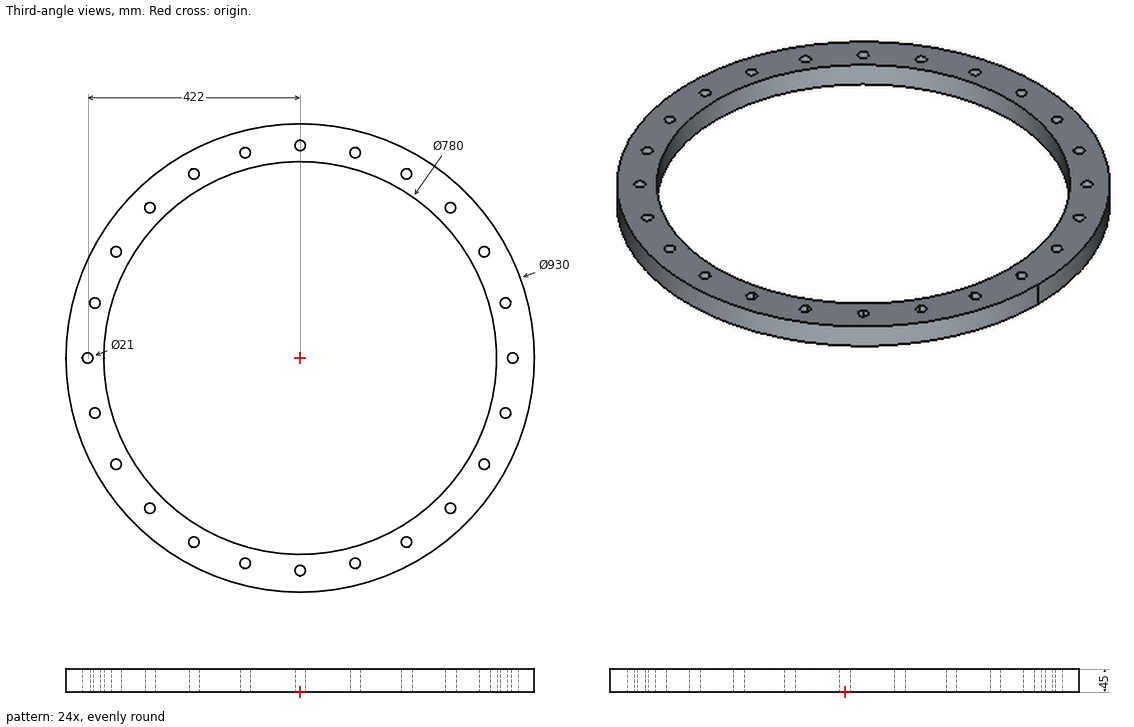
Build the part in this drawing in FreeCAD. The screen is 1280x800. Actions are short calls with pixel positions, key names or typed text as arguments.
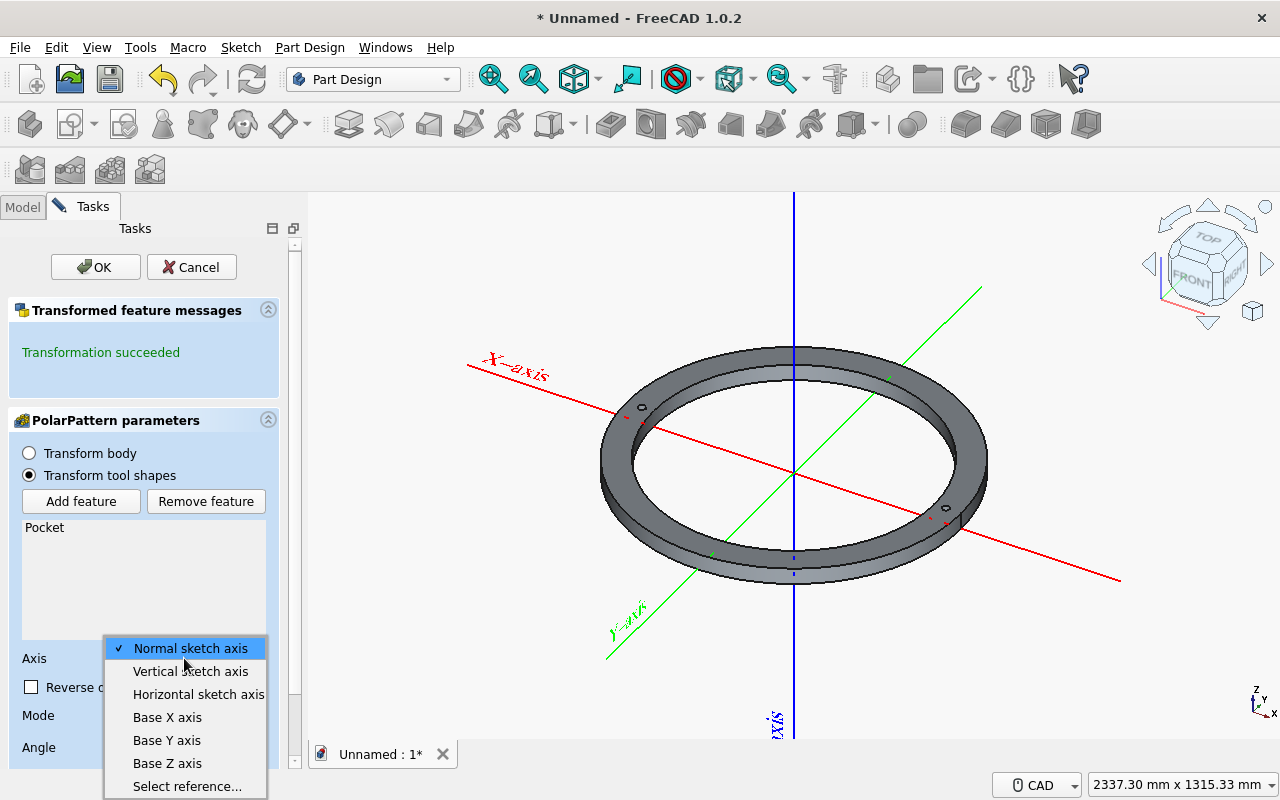
click(184, 764)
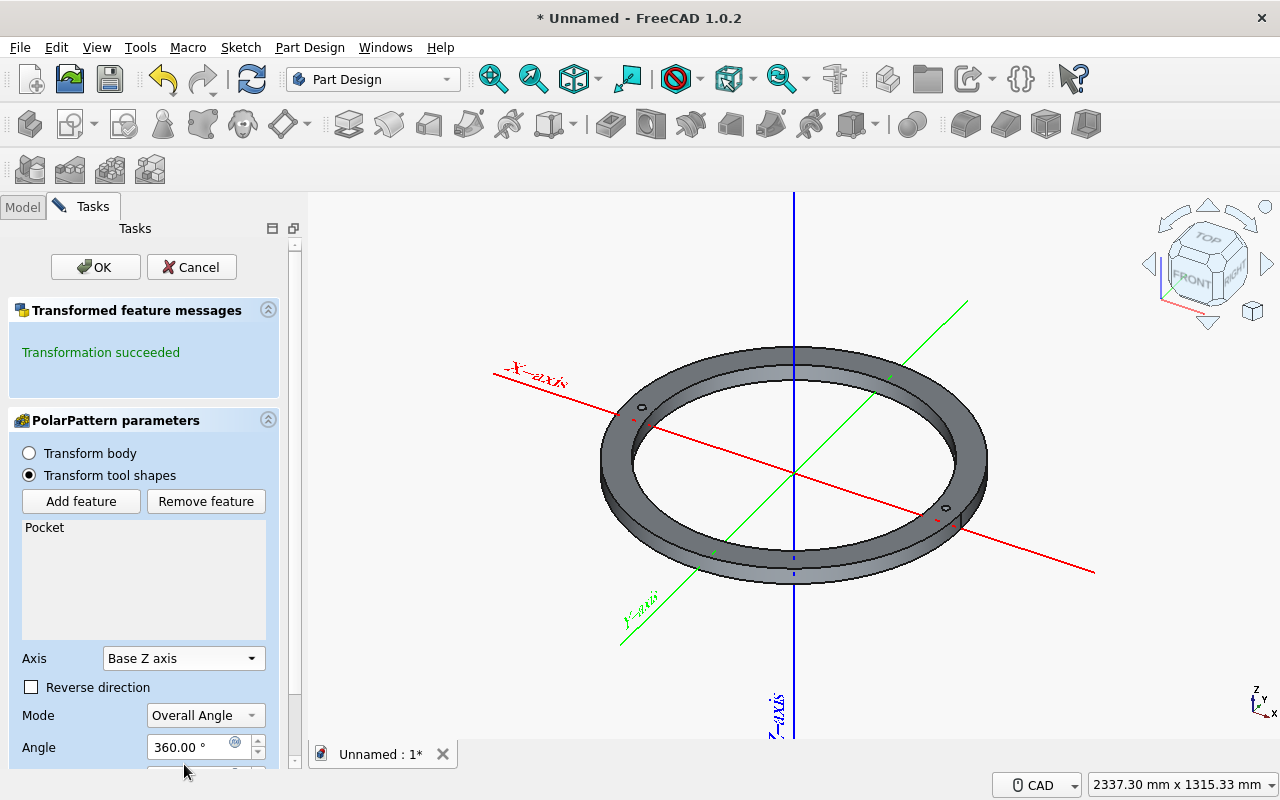
scroll(295, 503, down, 2)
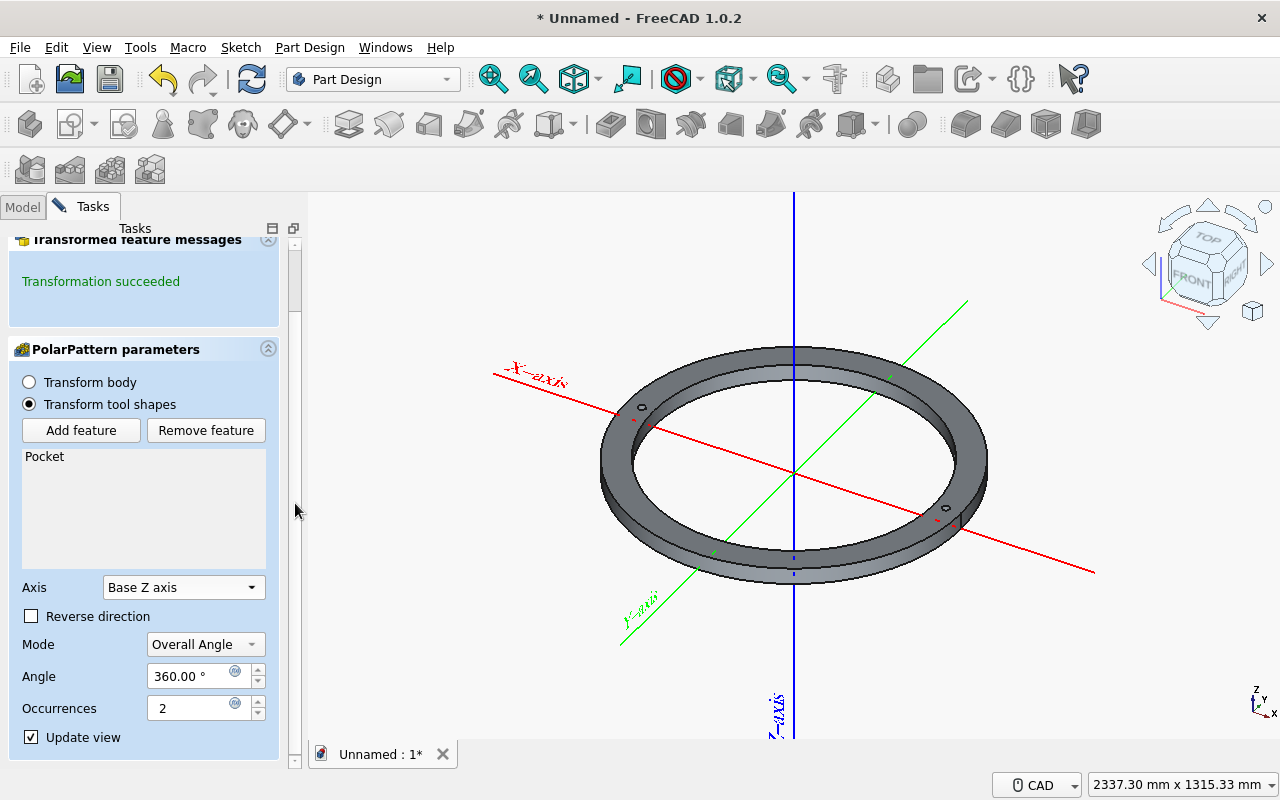
triple_click(198, 708)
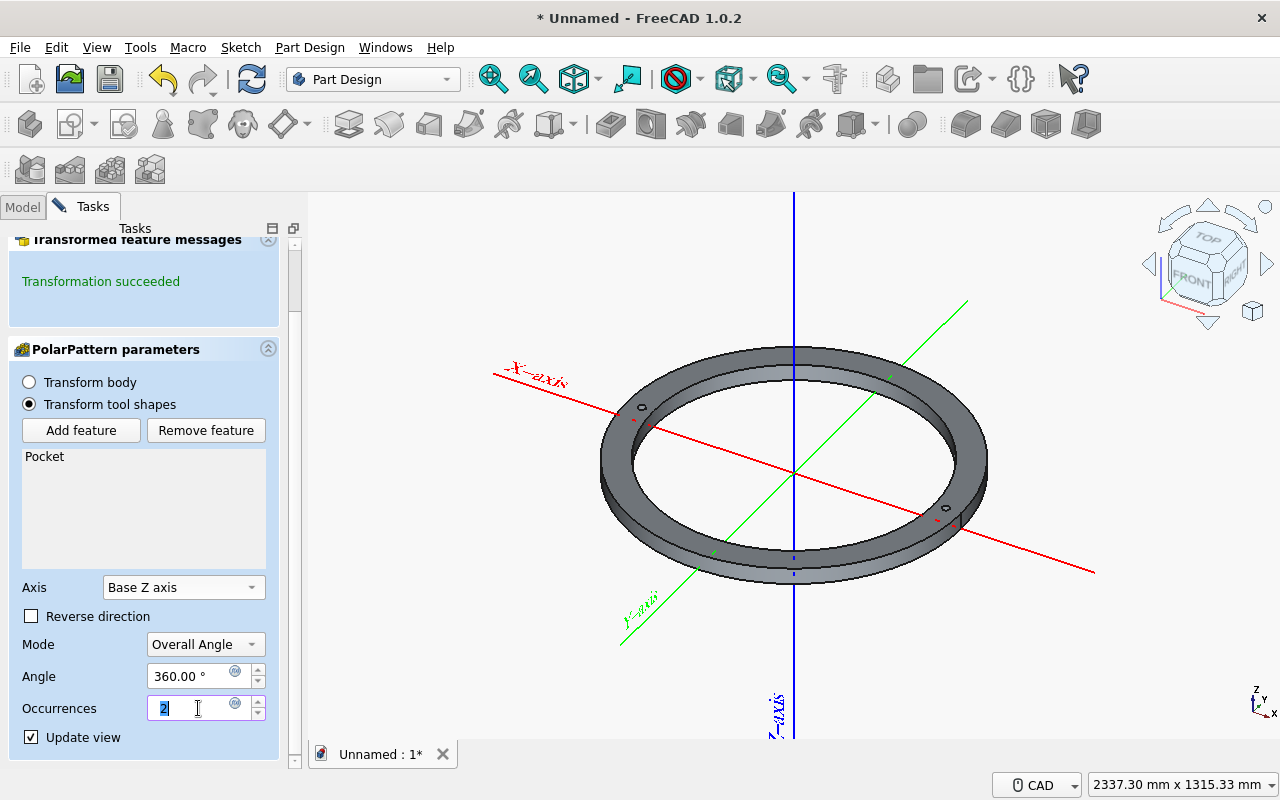
text(24)
key(Tab)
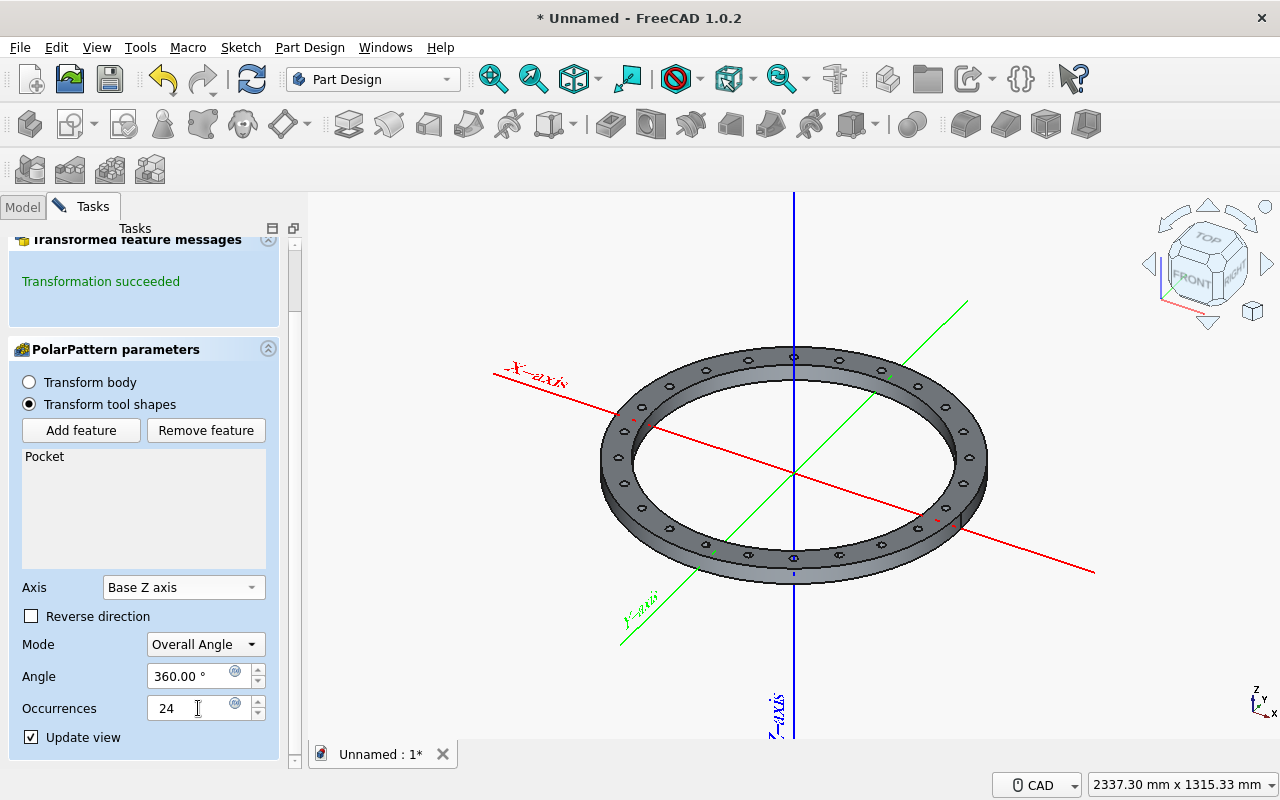
scroll(295, 503, up, 2)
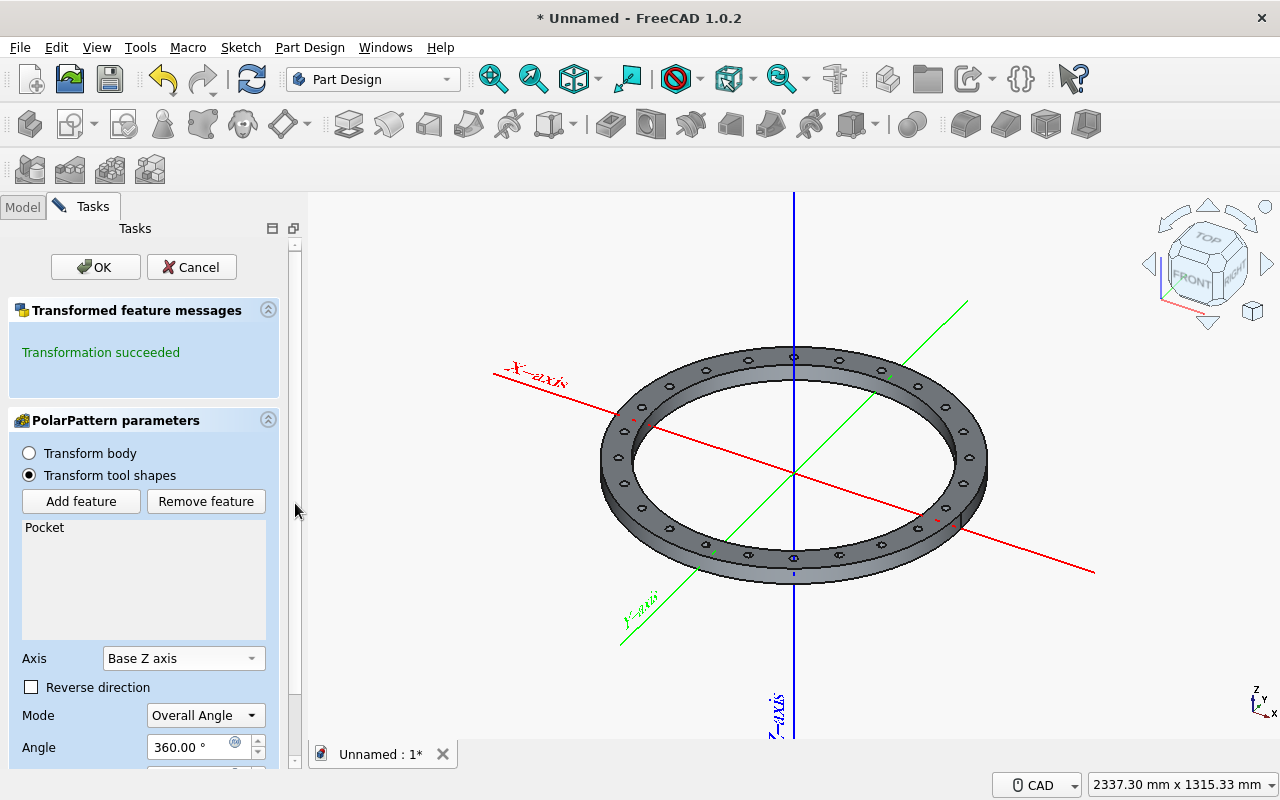
click(96, 267)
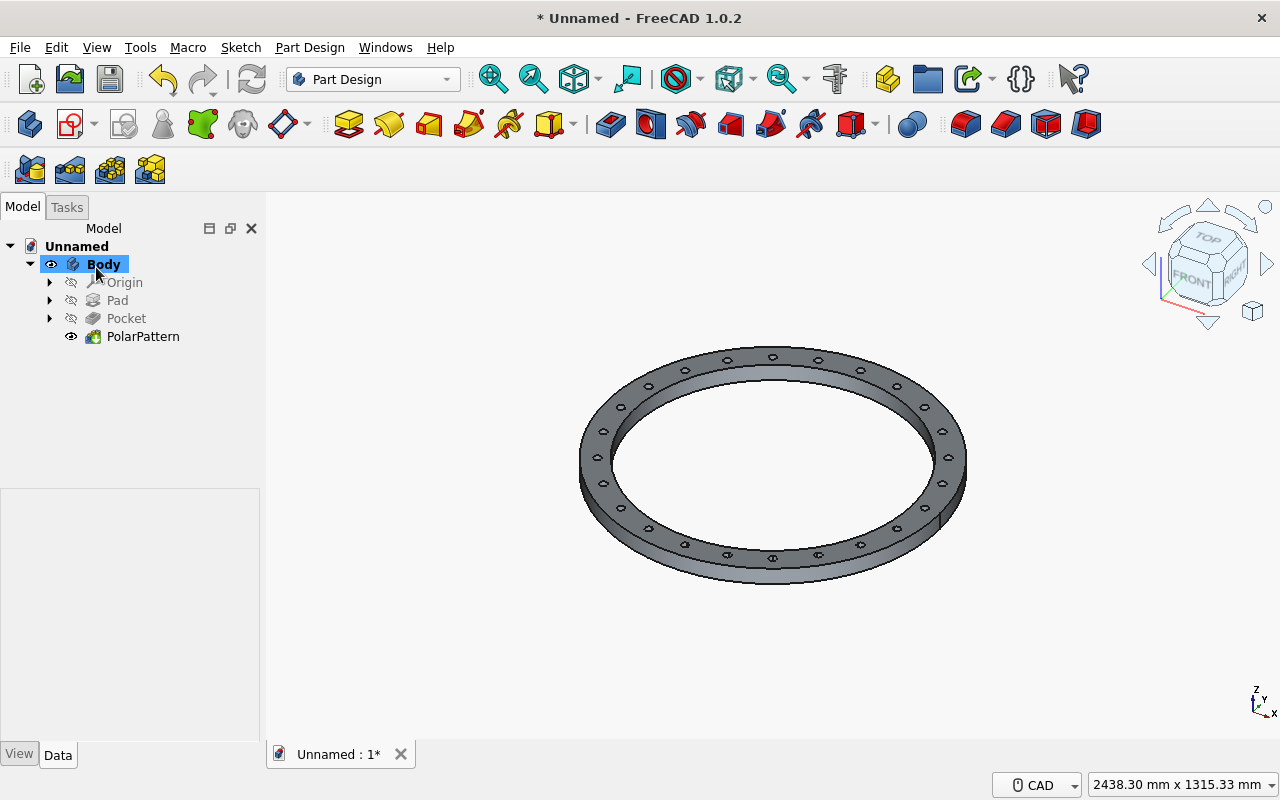
key(0)